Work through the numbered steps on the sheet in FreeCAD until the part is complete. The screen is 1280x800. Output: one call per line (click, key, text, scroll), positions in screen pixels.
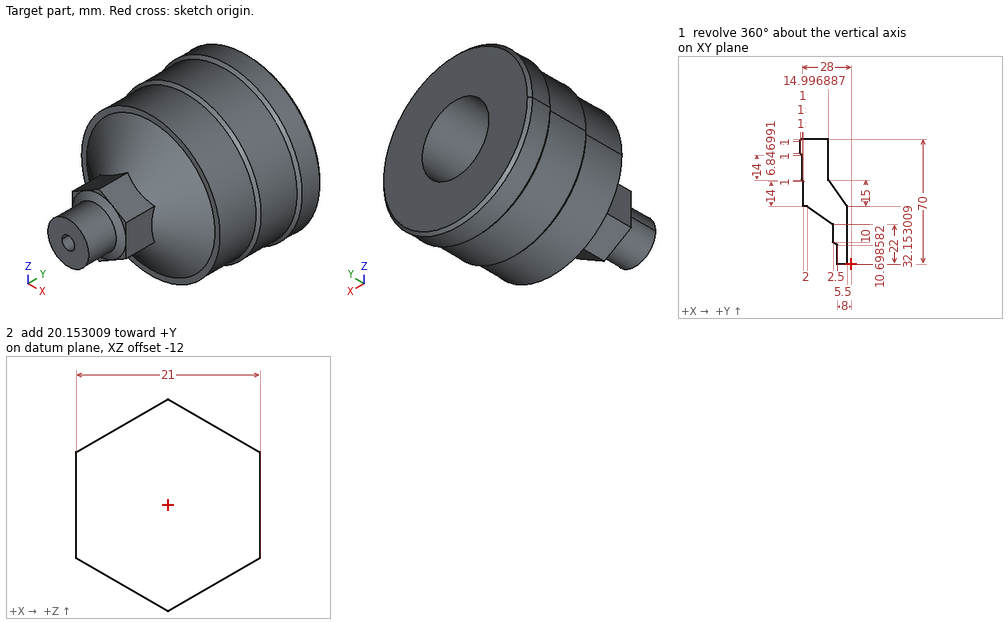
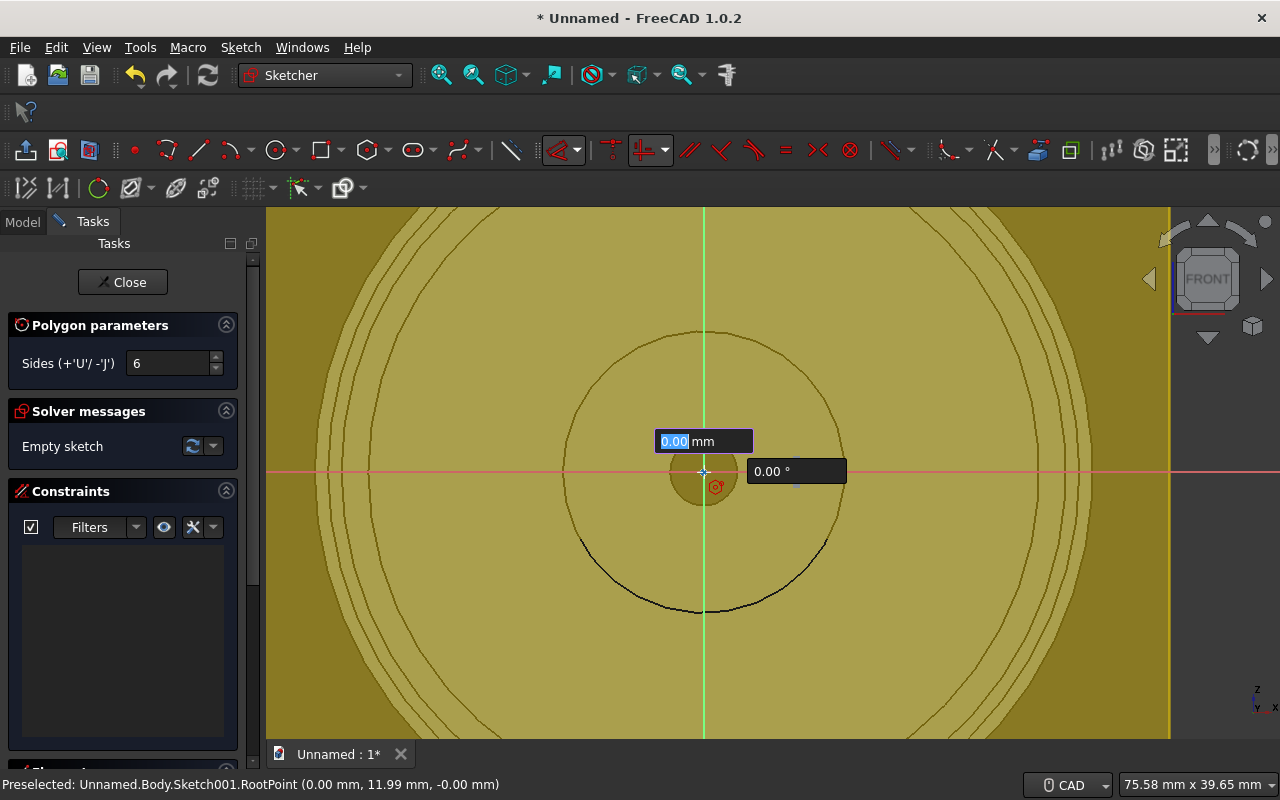
click(704, 635)
key(Escape)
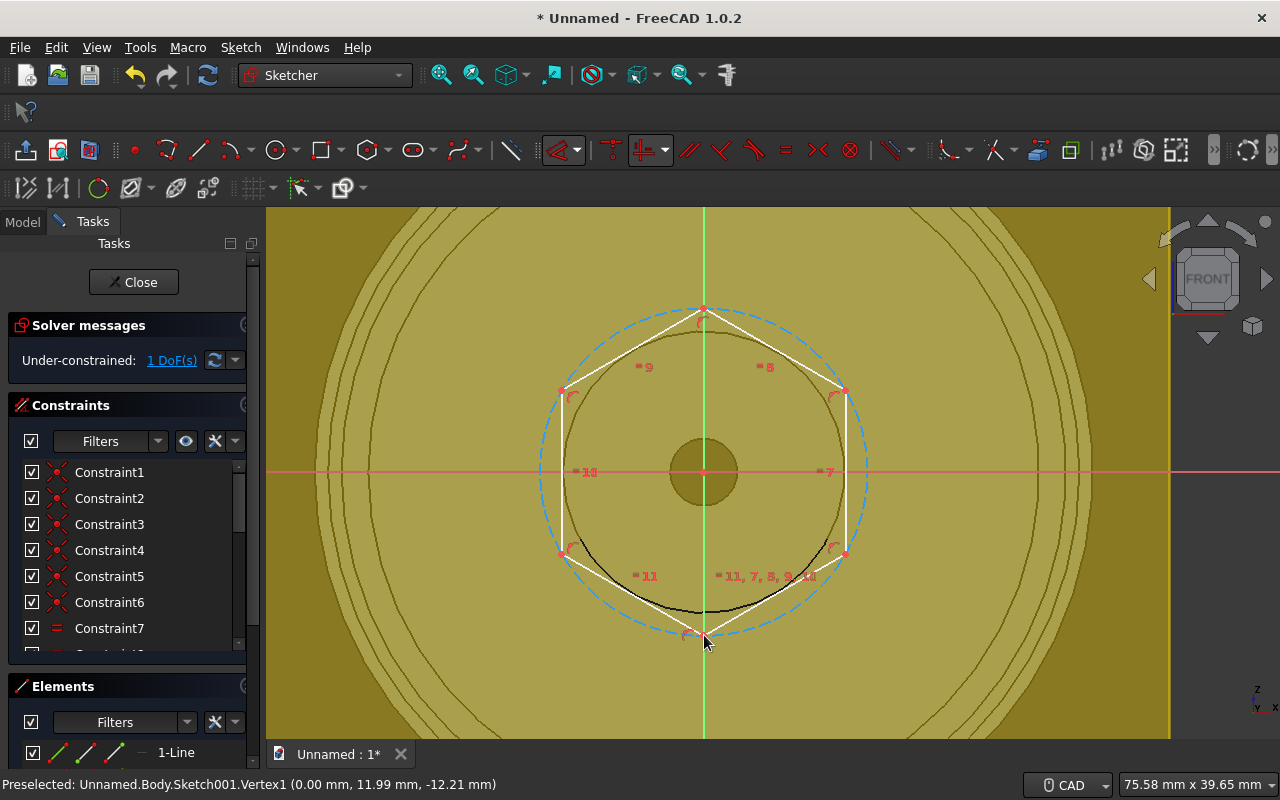
click(562, 390)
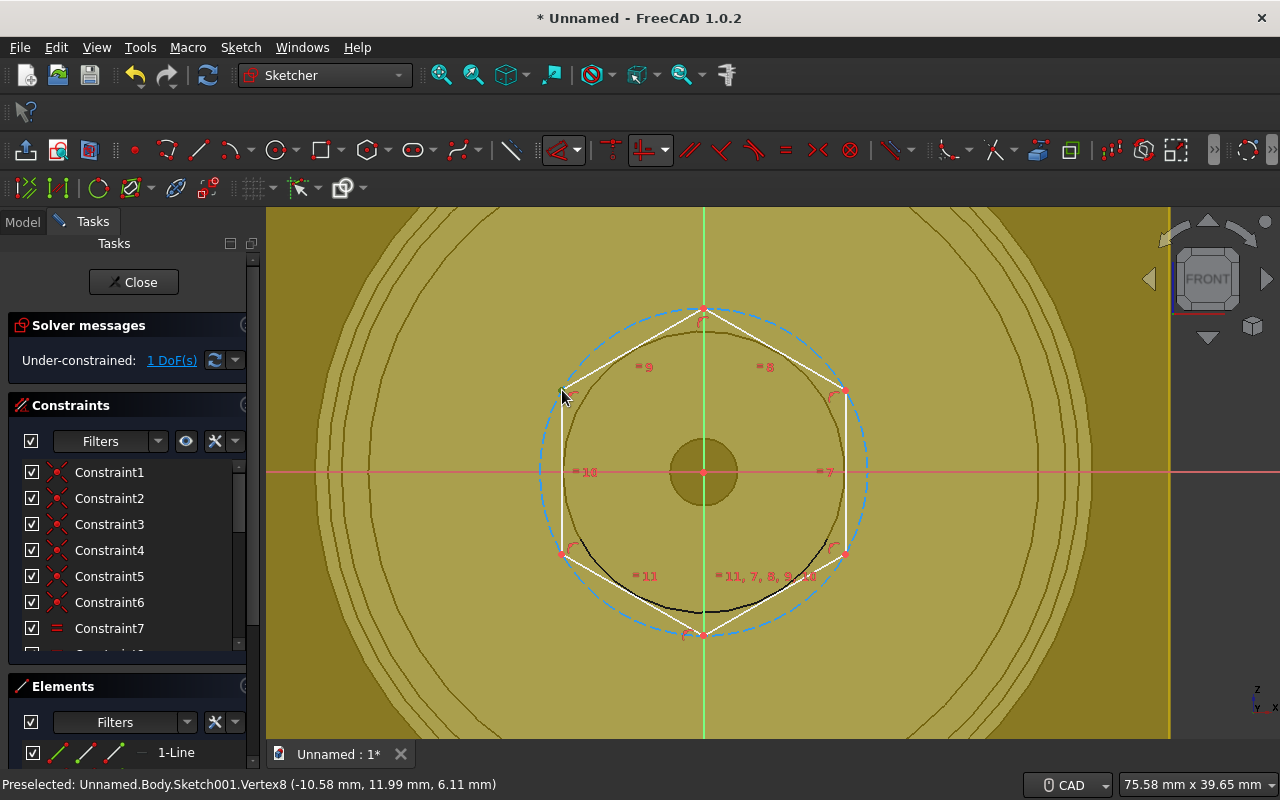
click(846, 554)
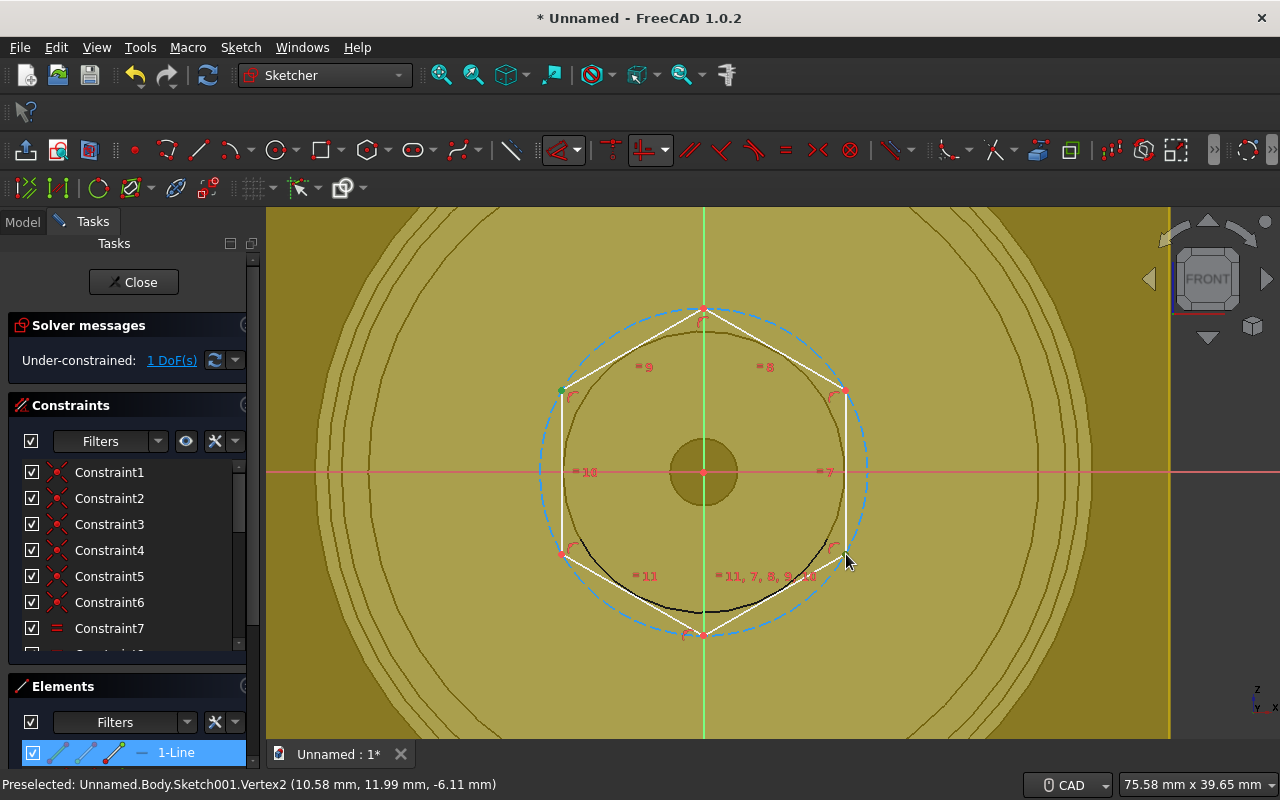
key(l)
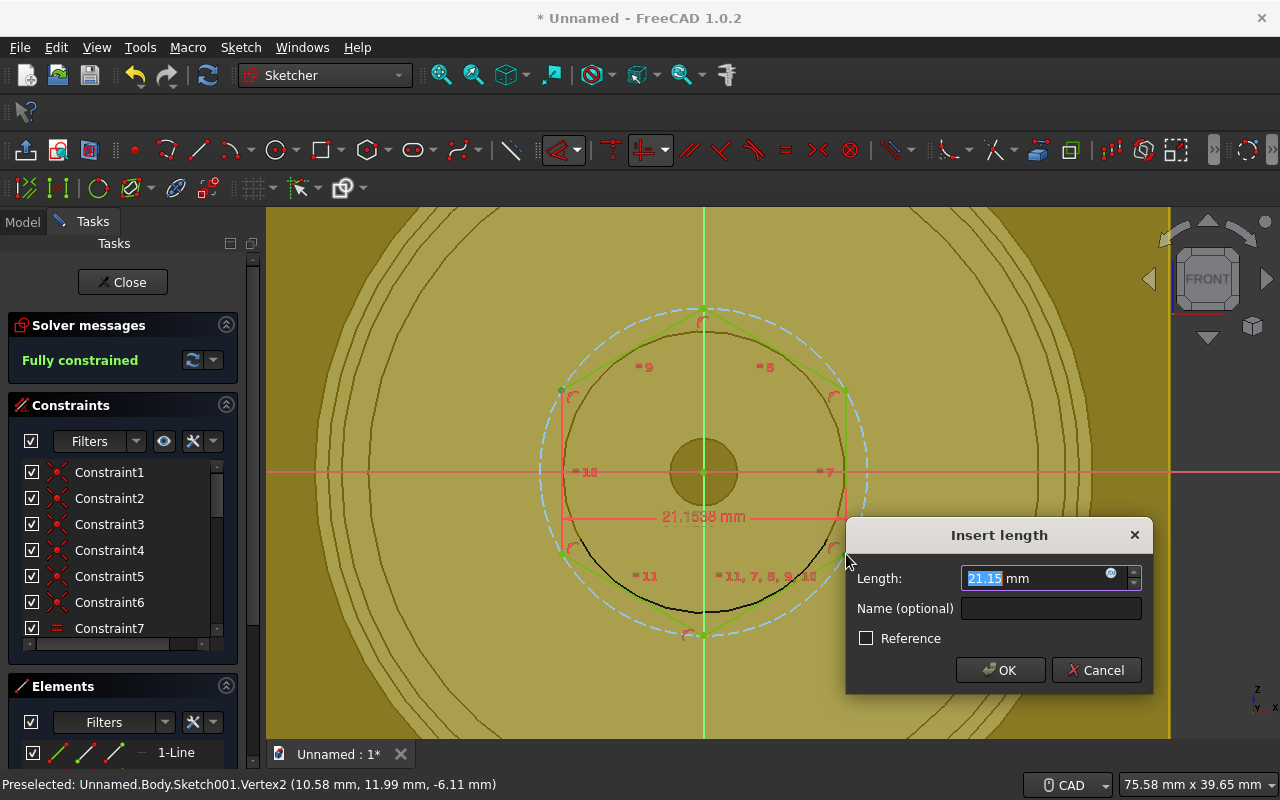
text(21)
key(Return)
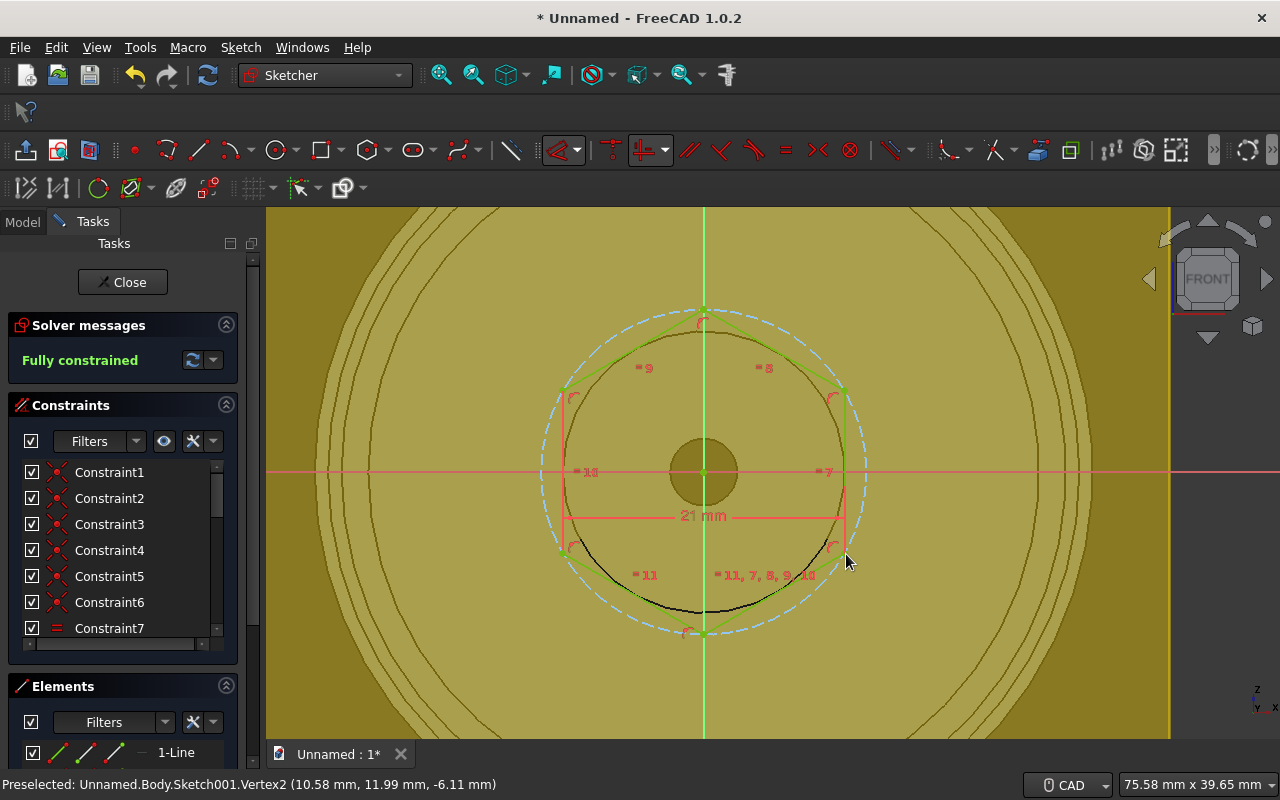
click(123, 282)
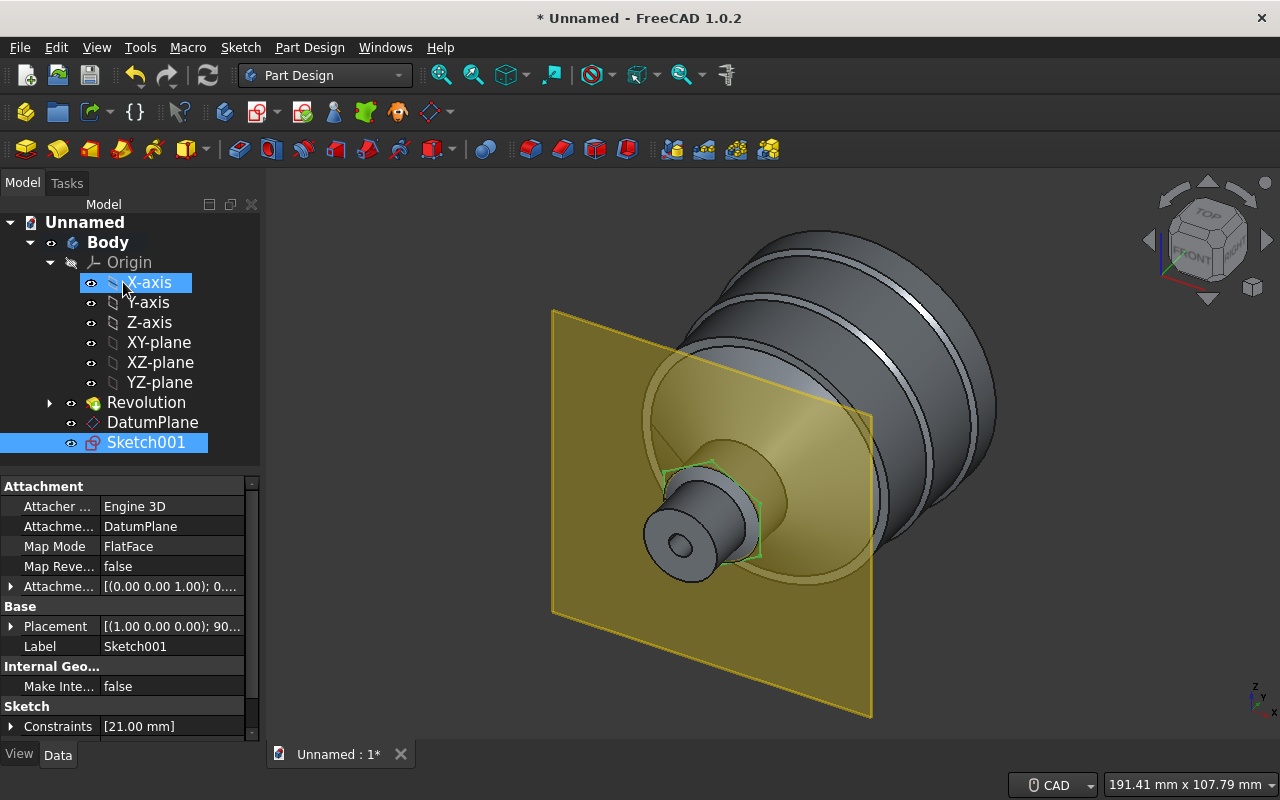
click(26, 150)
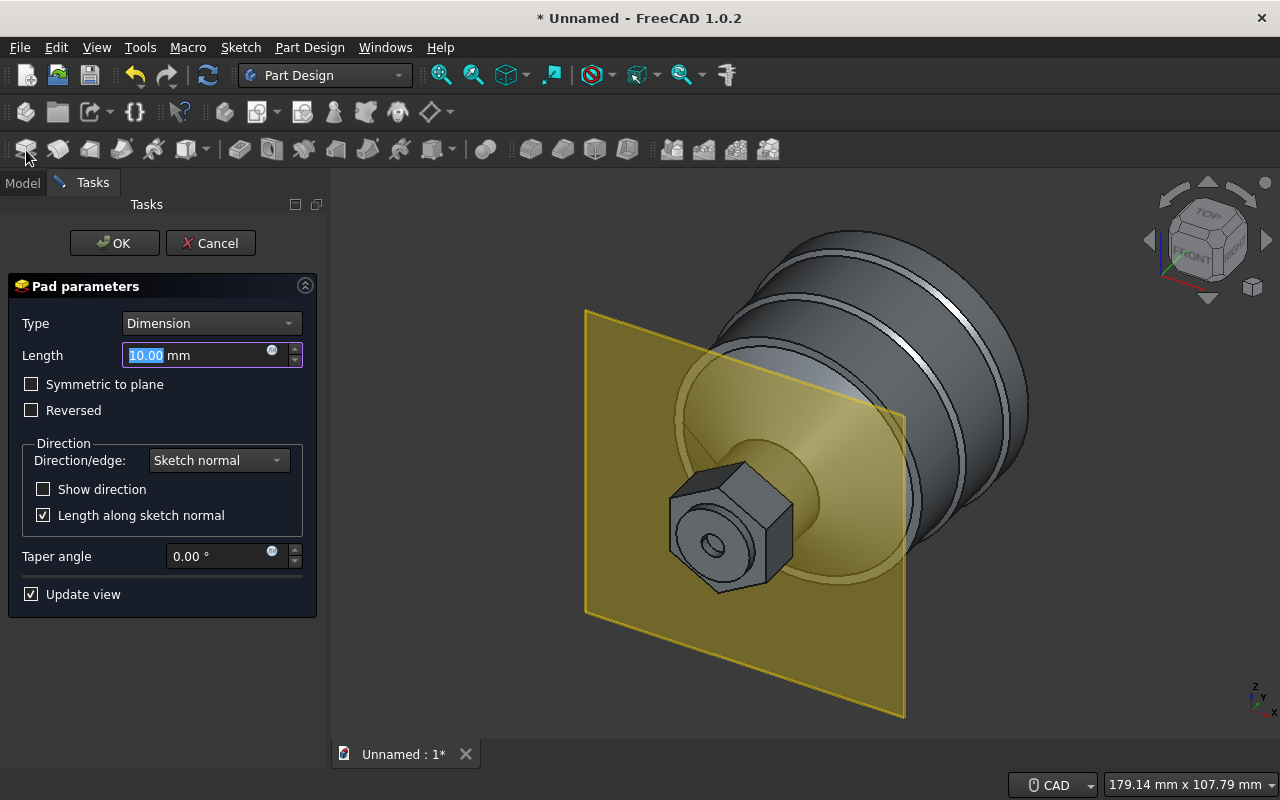
text(20.153009)
key(Tab)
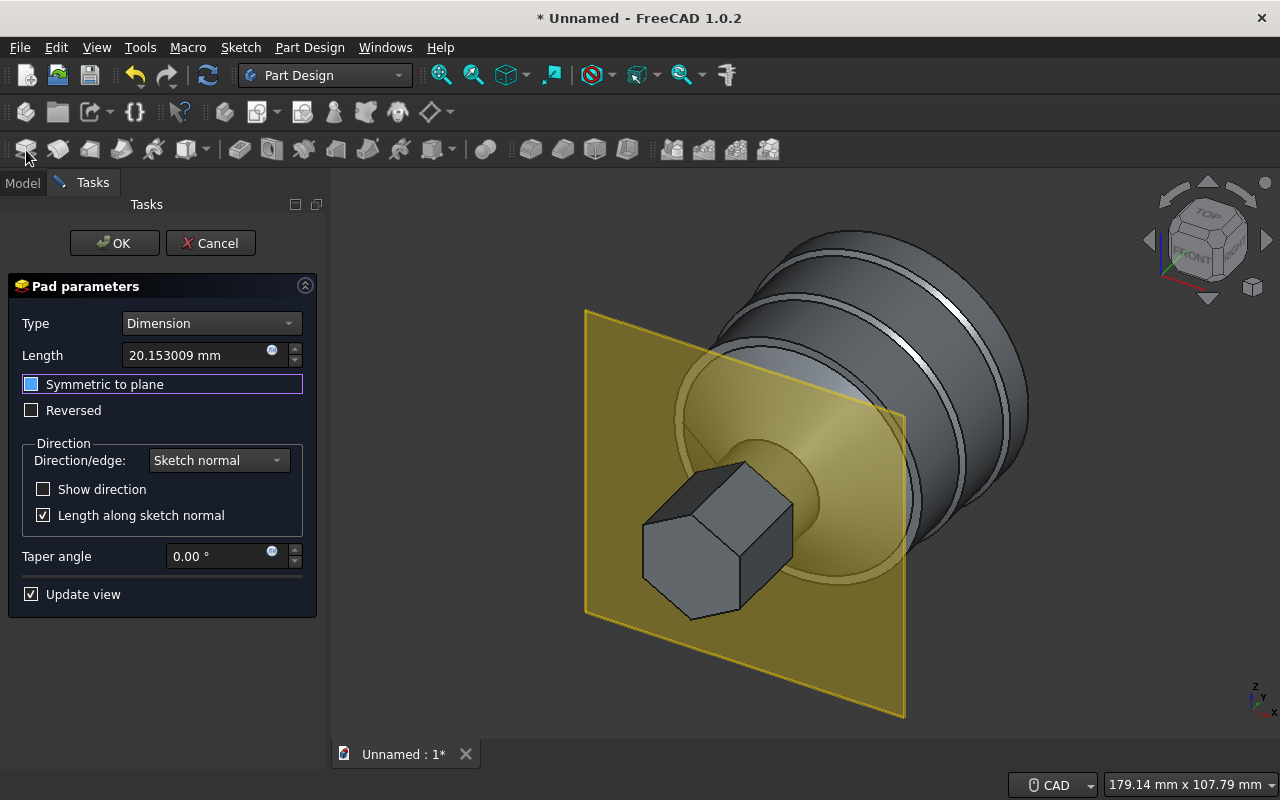
click(30, 410)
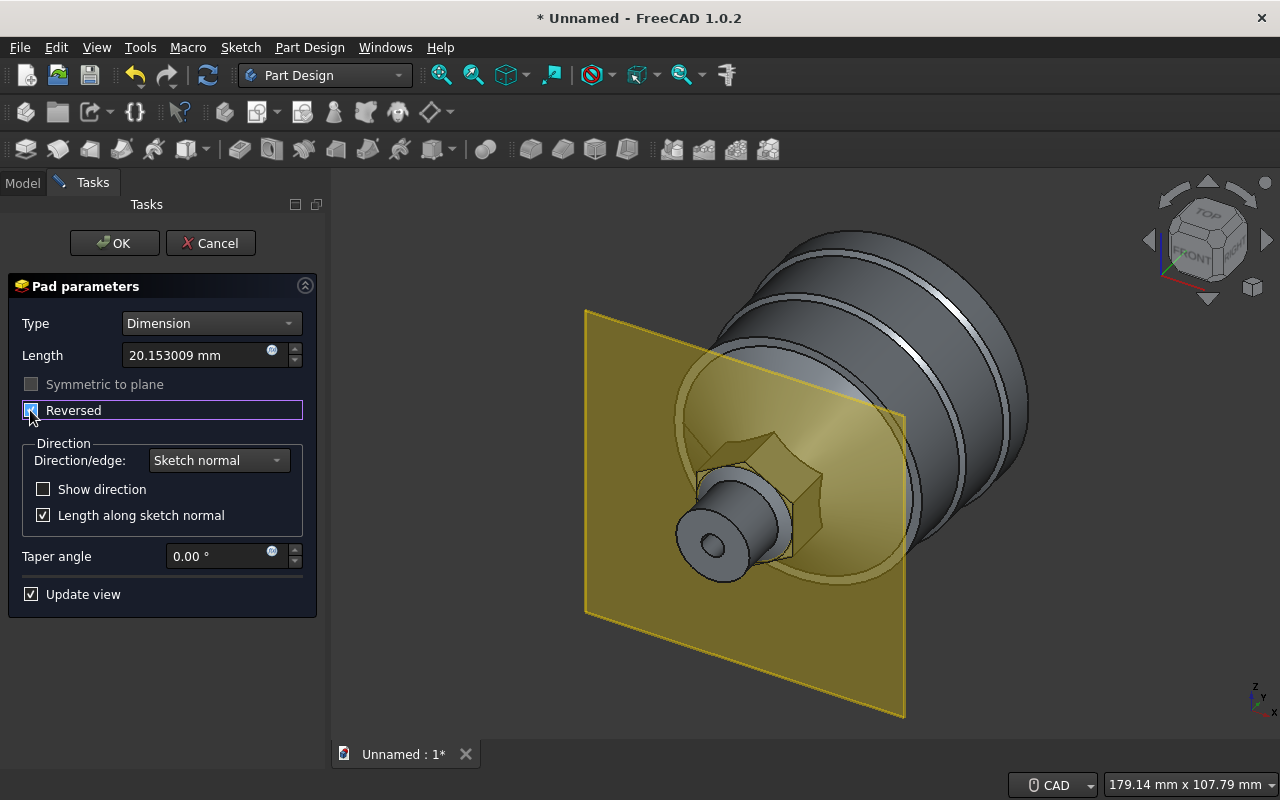
click(115, 243)